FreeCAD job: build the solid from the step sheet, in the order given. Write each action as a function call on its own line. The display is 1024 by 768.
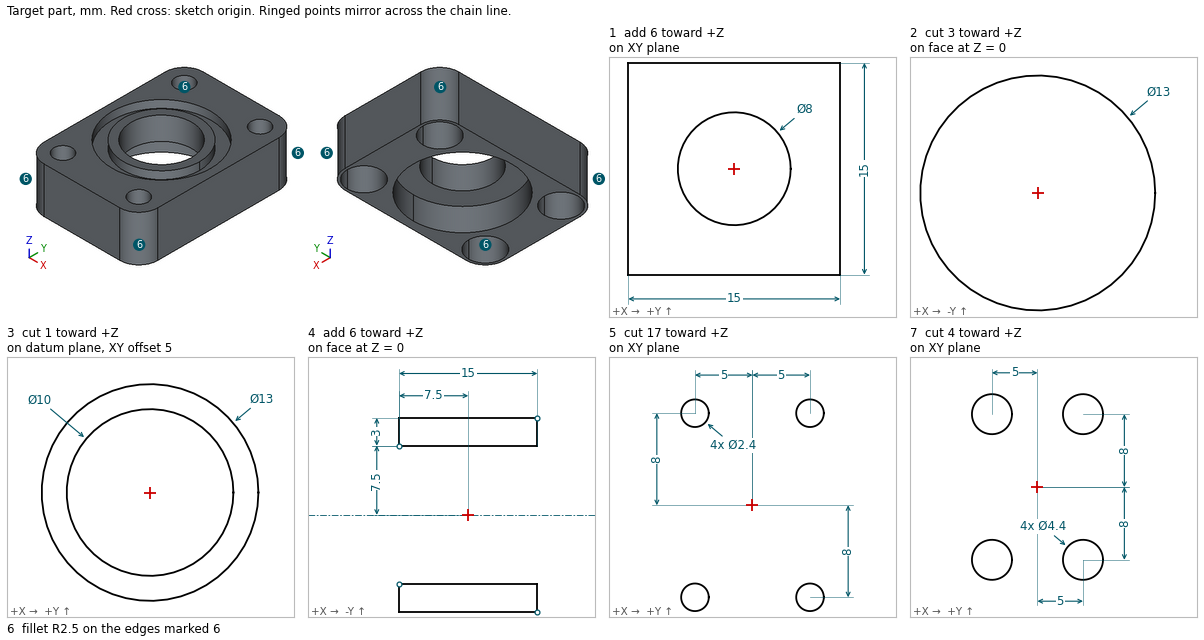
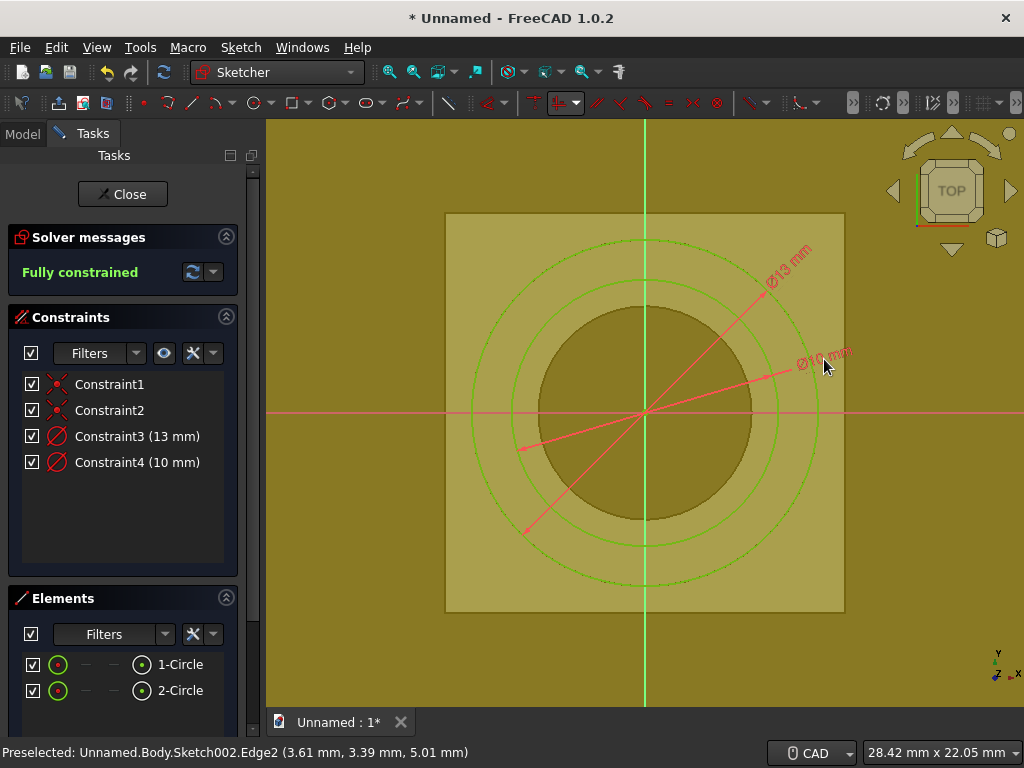
click(123, 194)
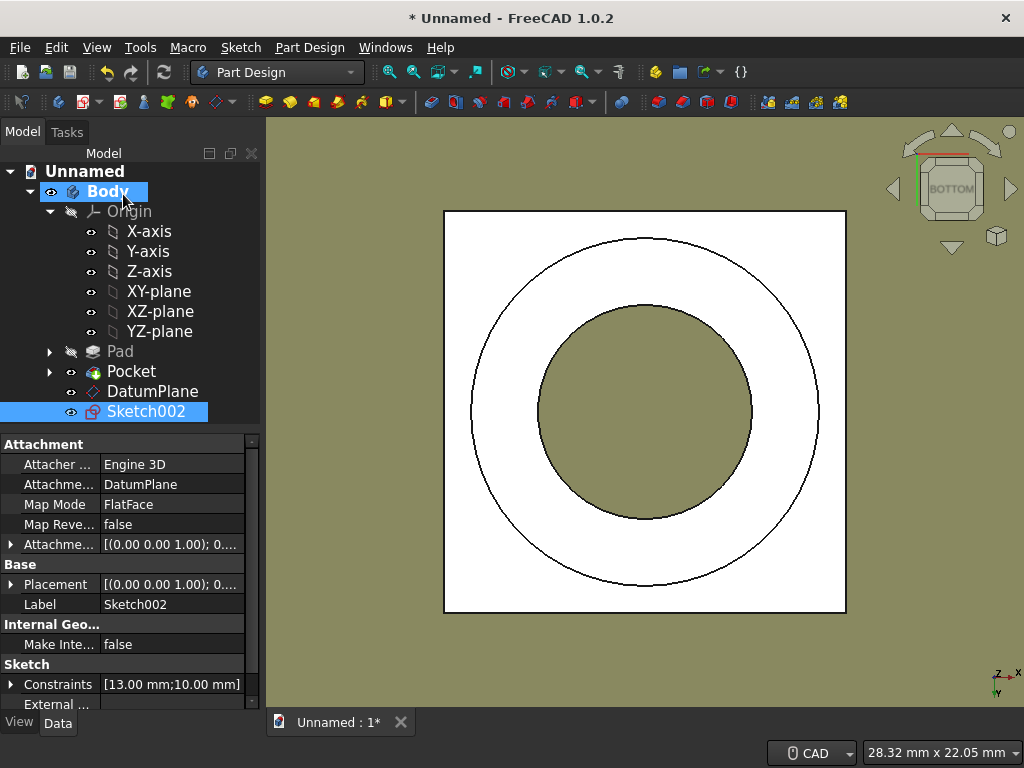
click(432, 102)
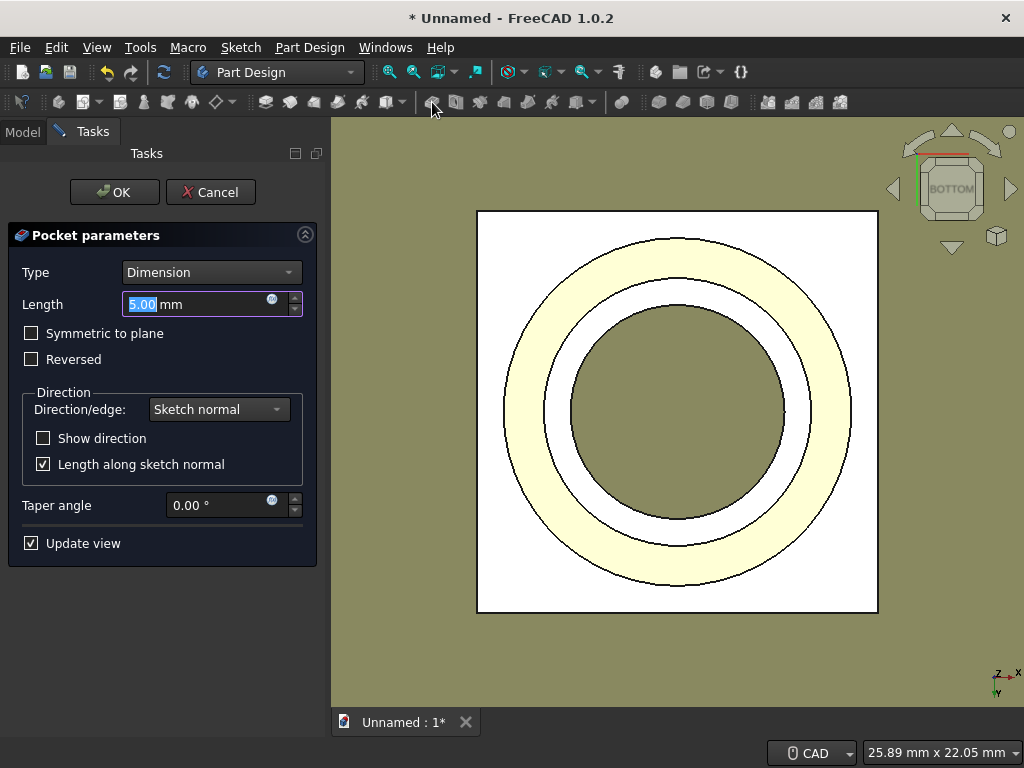
text(1)
key(Tab)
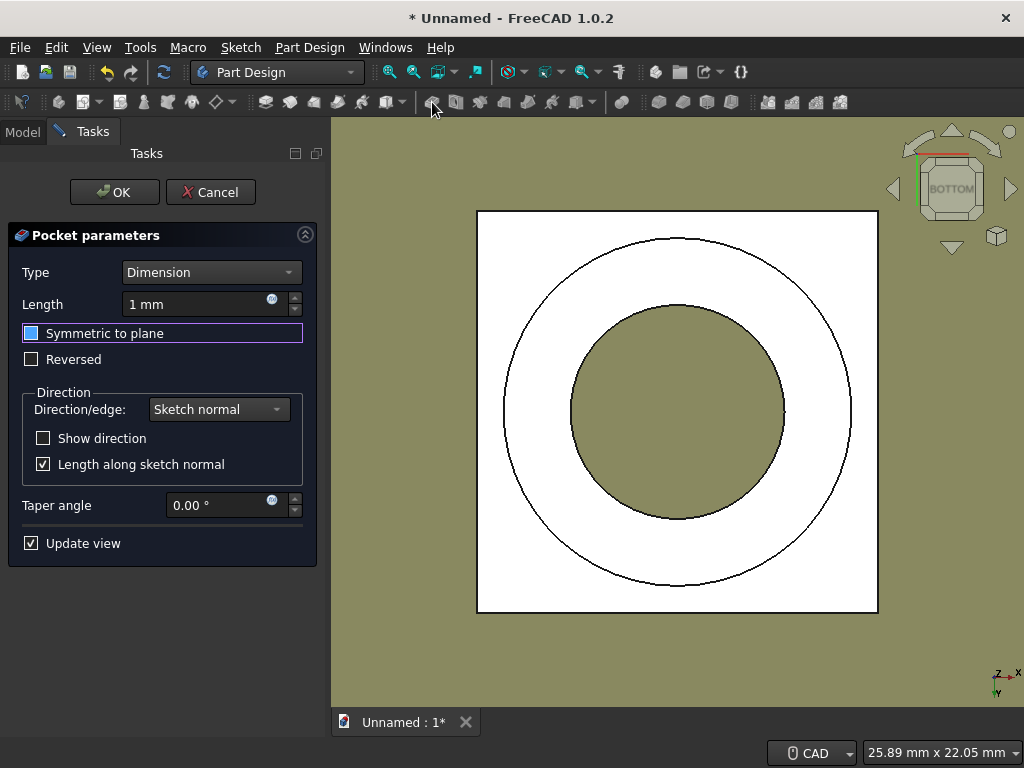
click(30, 359)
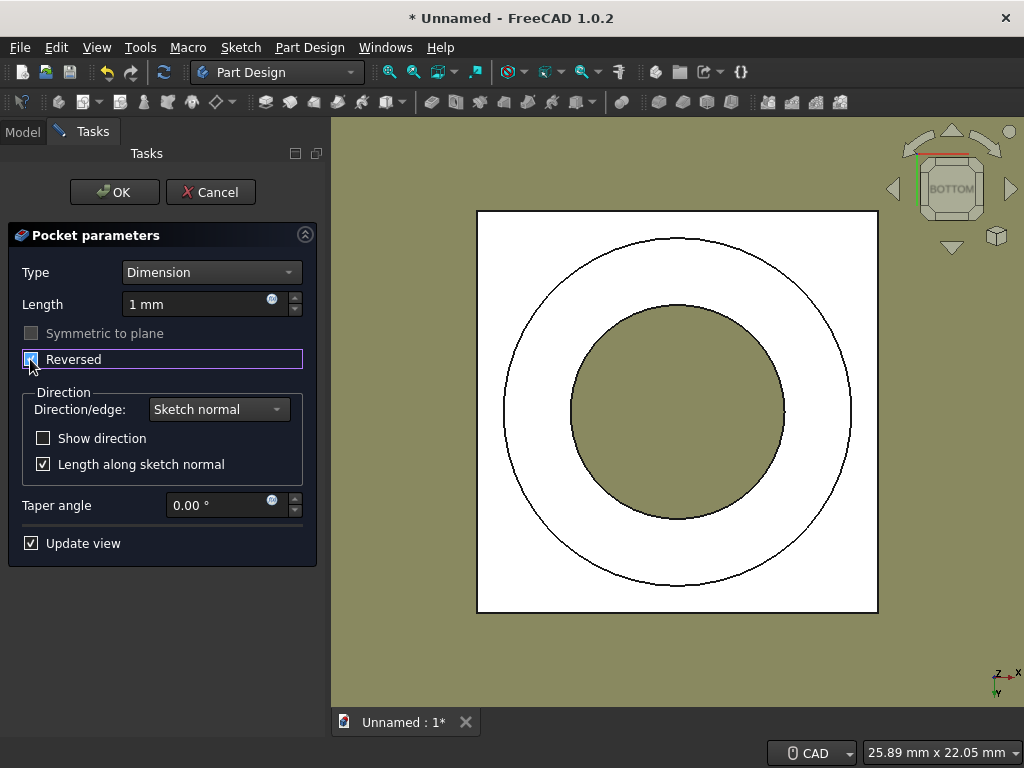
click(115, 192)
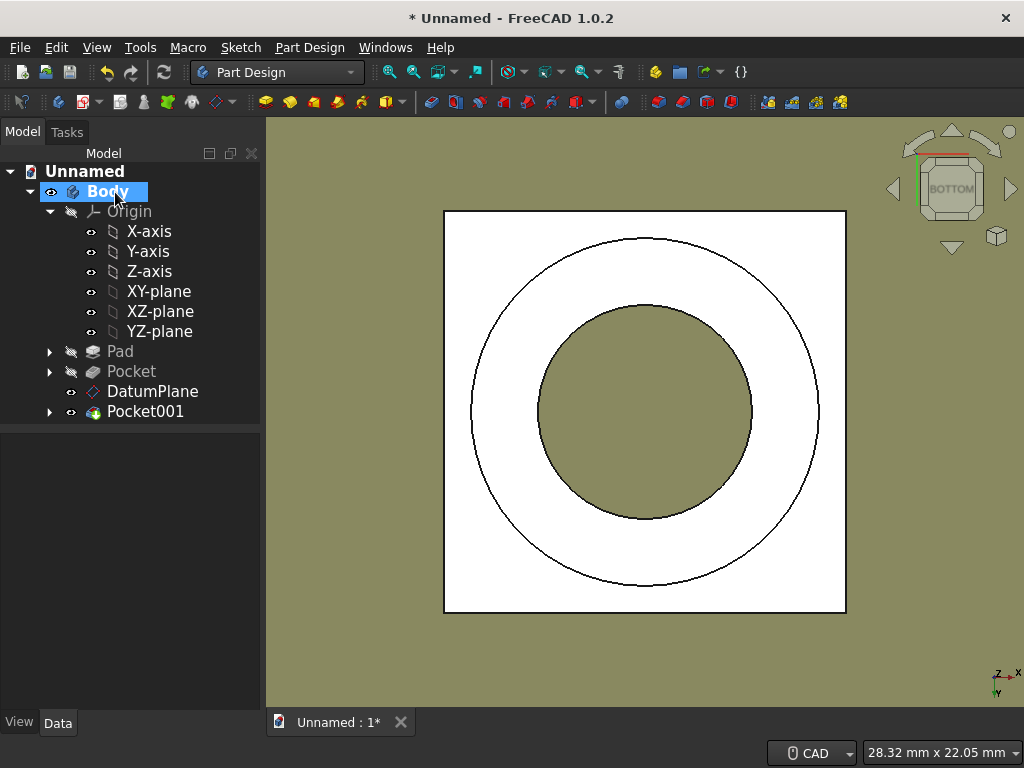
click(116, 392)
key(space)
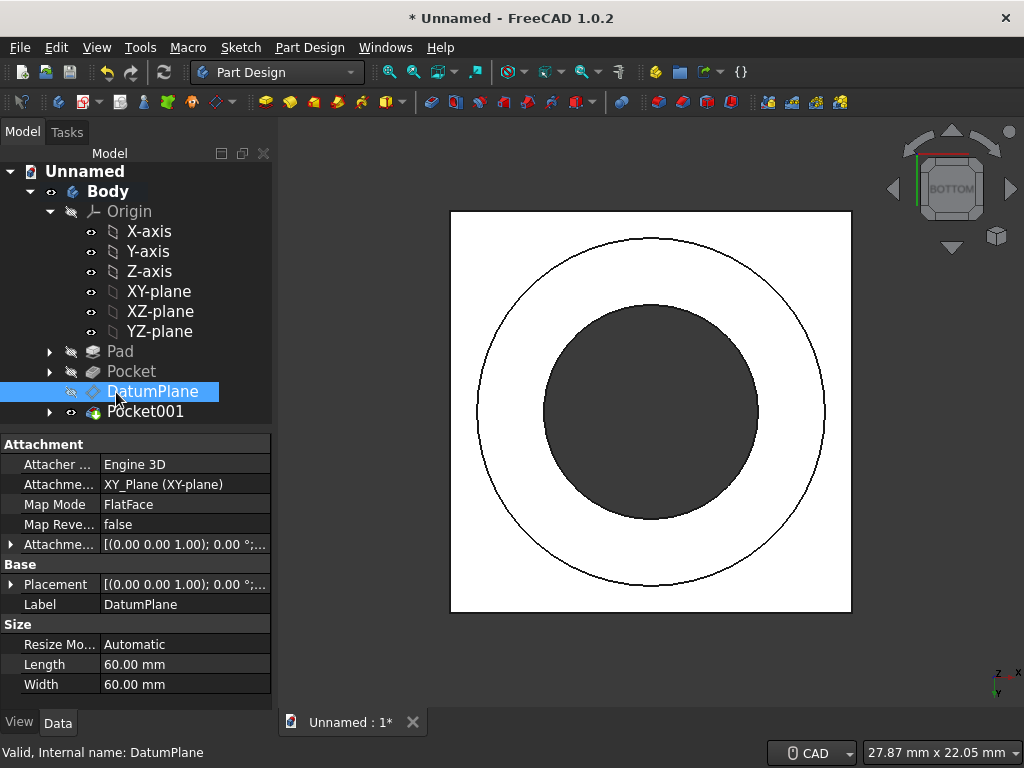
click(823, 583)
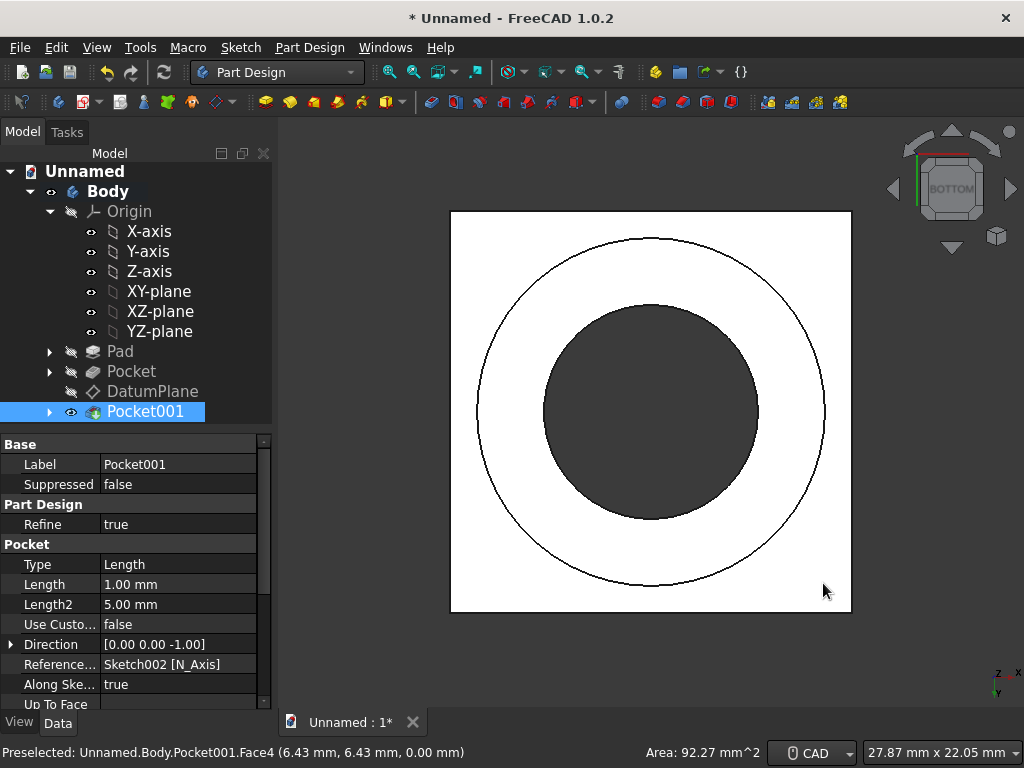
click(84, 102)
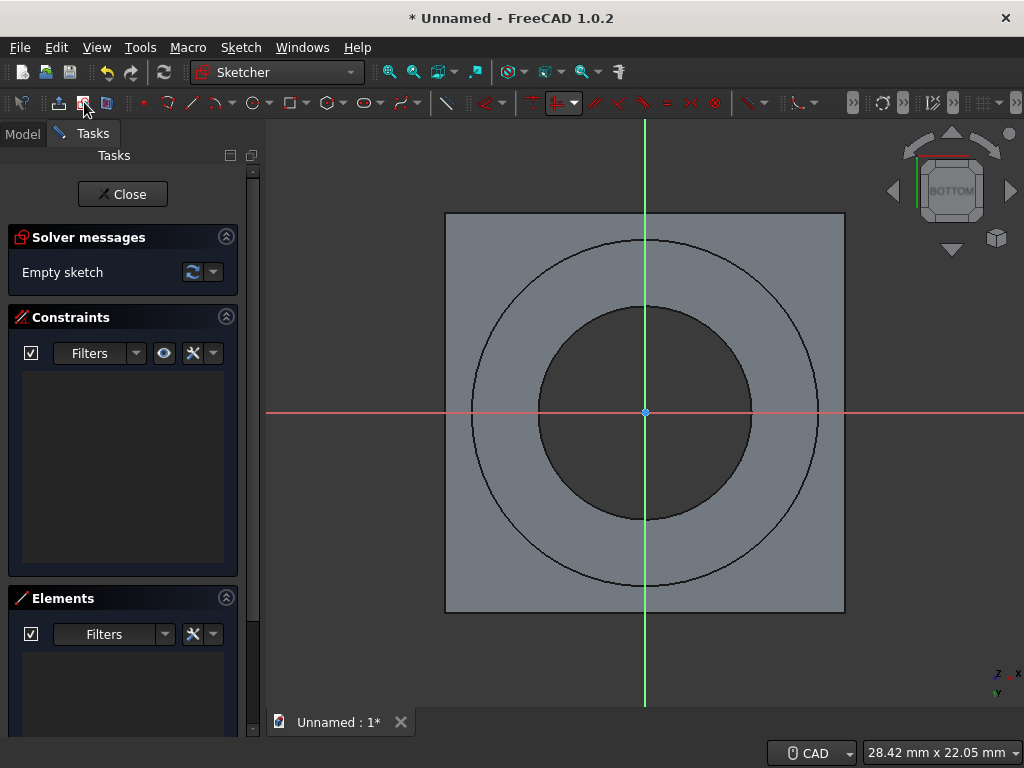
scroll(437, 413, down, 2)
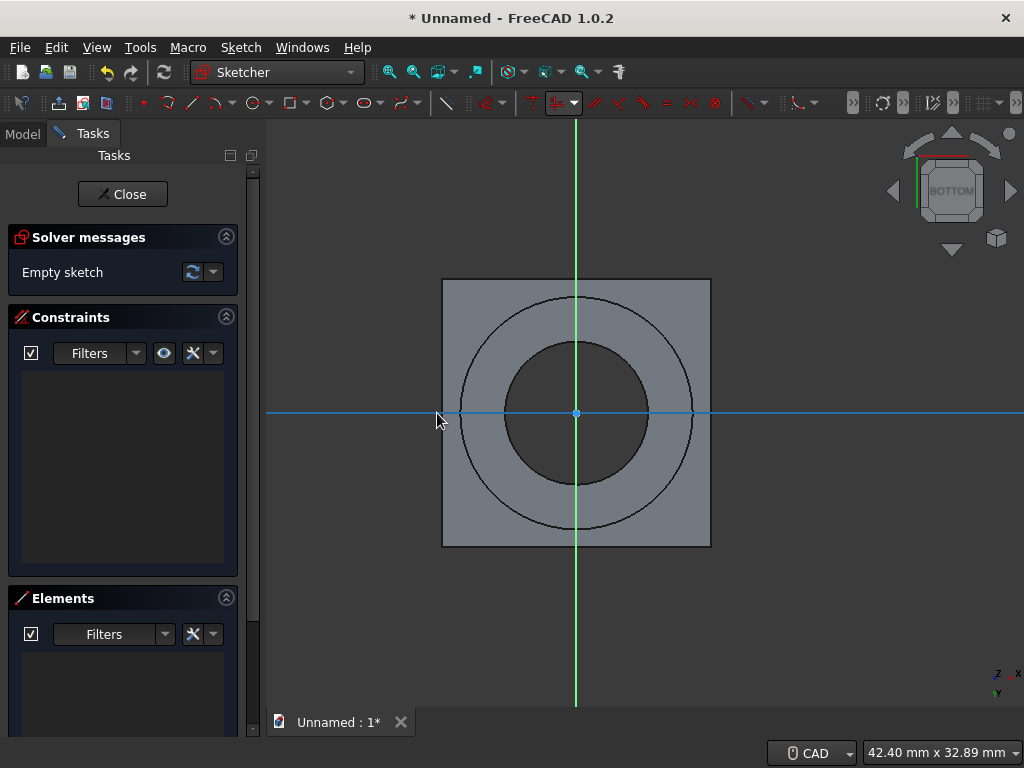
click(290, 104)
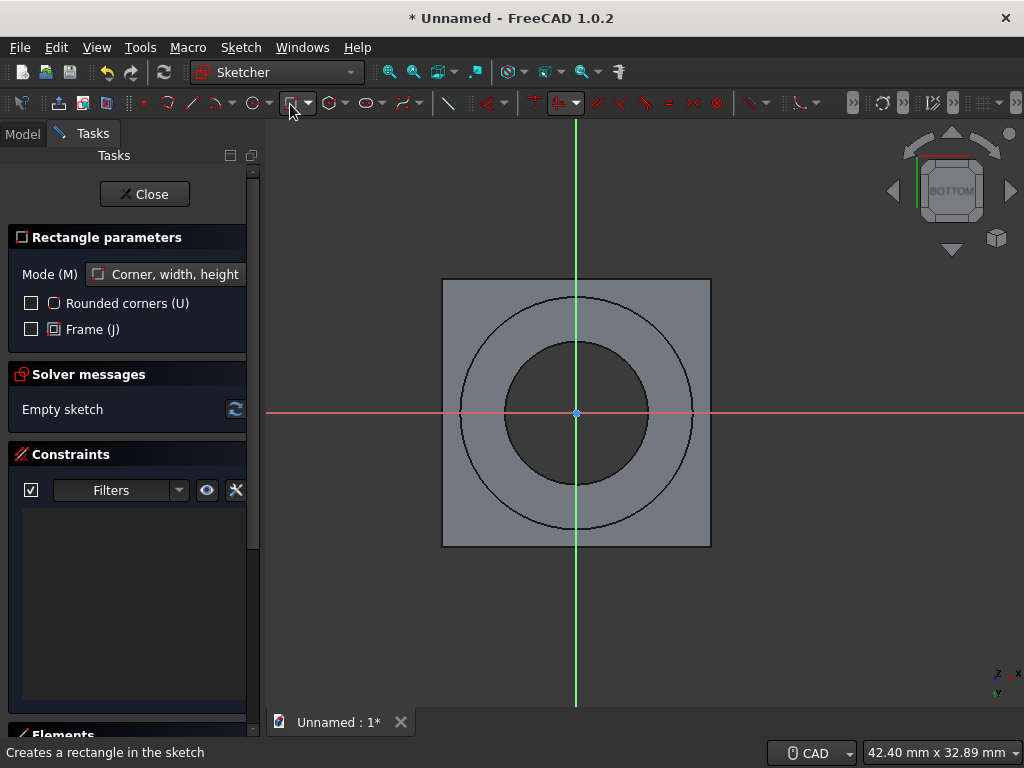
click(442, 225)
click(711, 279)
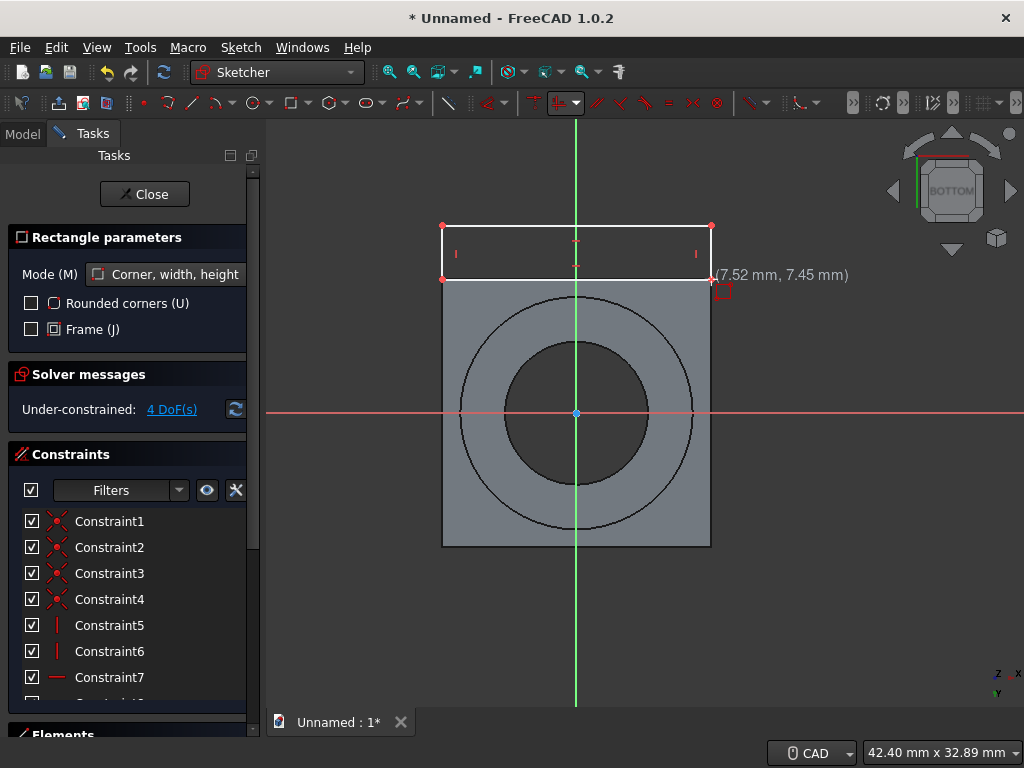
click(442, 547)
click(711, 601)
key(Escape)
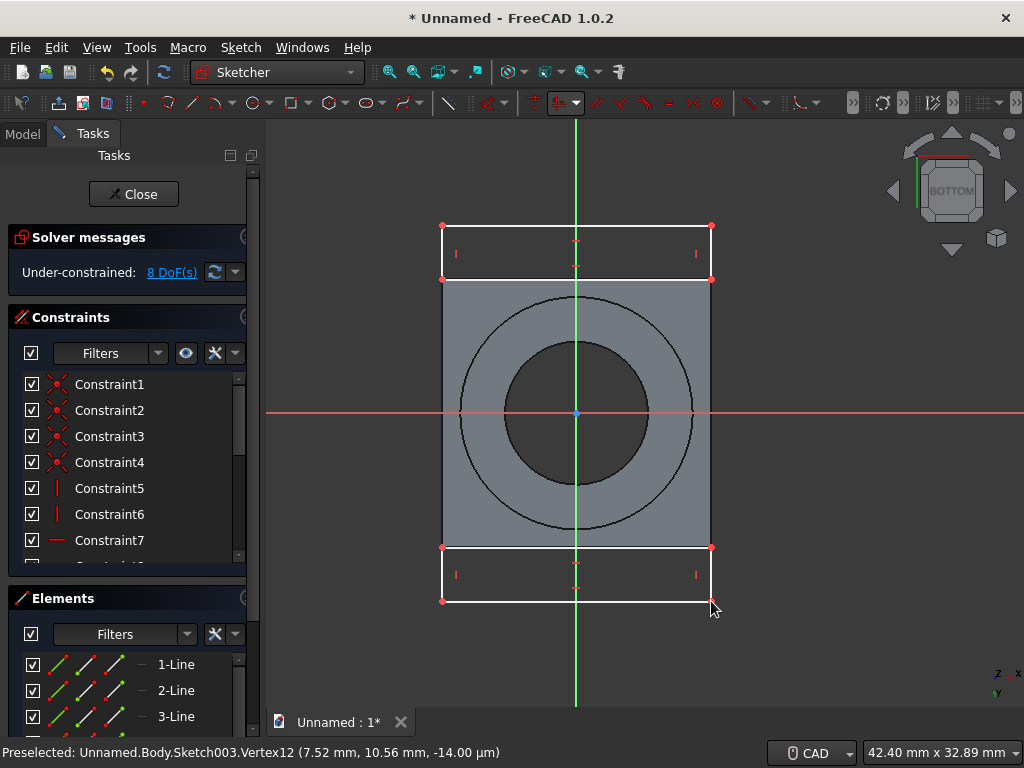
click(442, 280)